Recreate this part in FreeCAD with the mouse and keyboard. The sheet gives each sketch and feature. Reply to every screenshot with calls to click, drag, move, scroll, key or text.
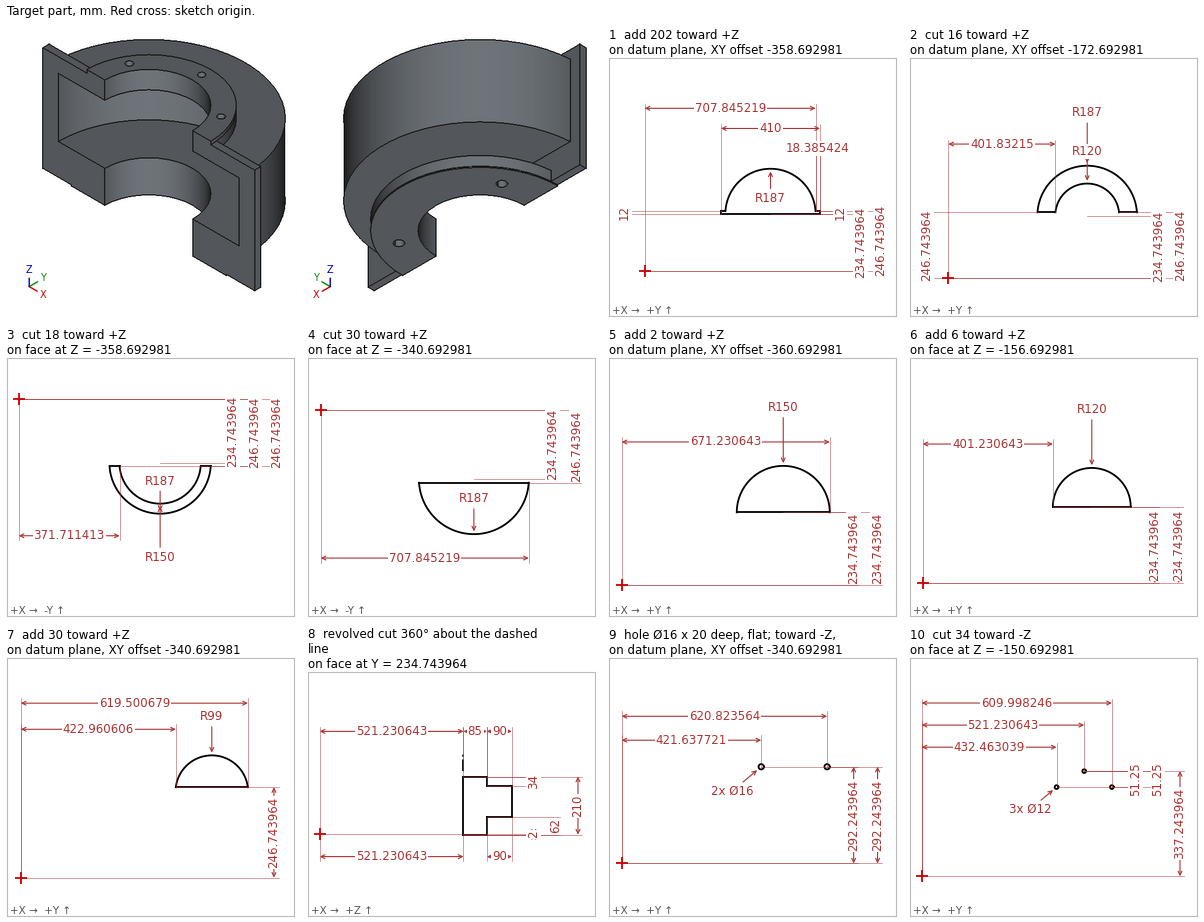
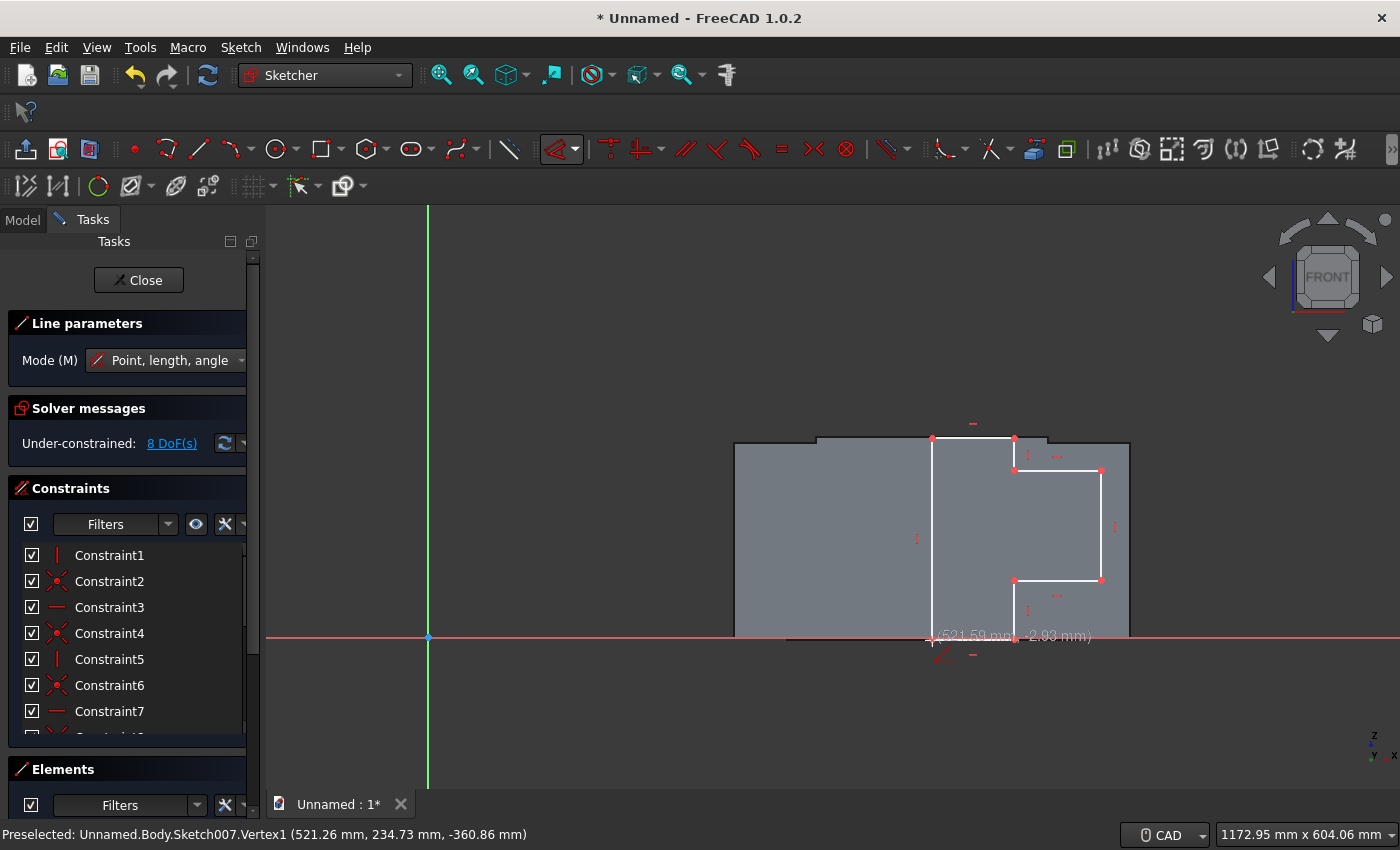
click(932, 417)
click(932, 356)
key(Escape)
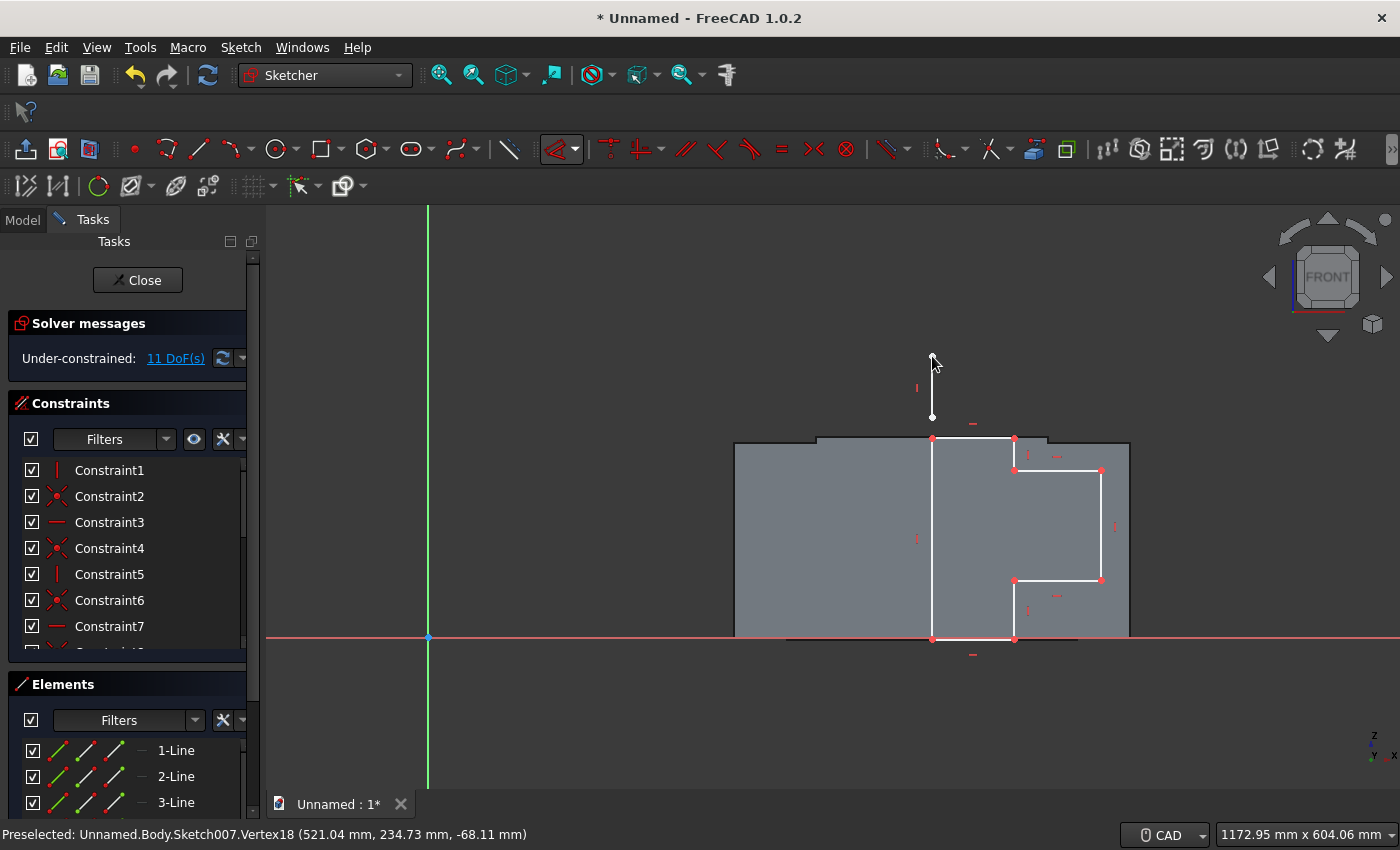
click(932, 400)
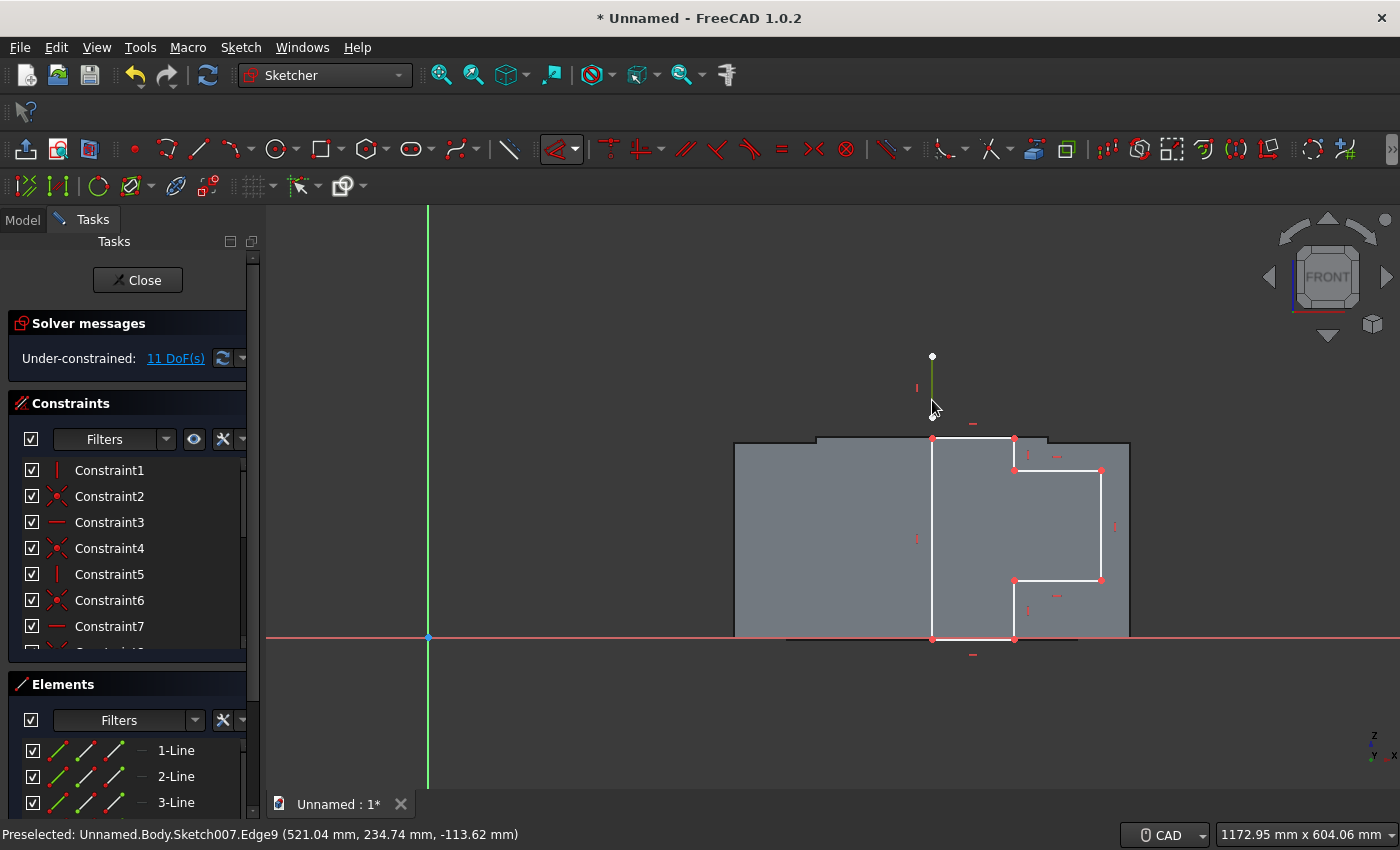
key(g)
key(n)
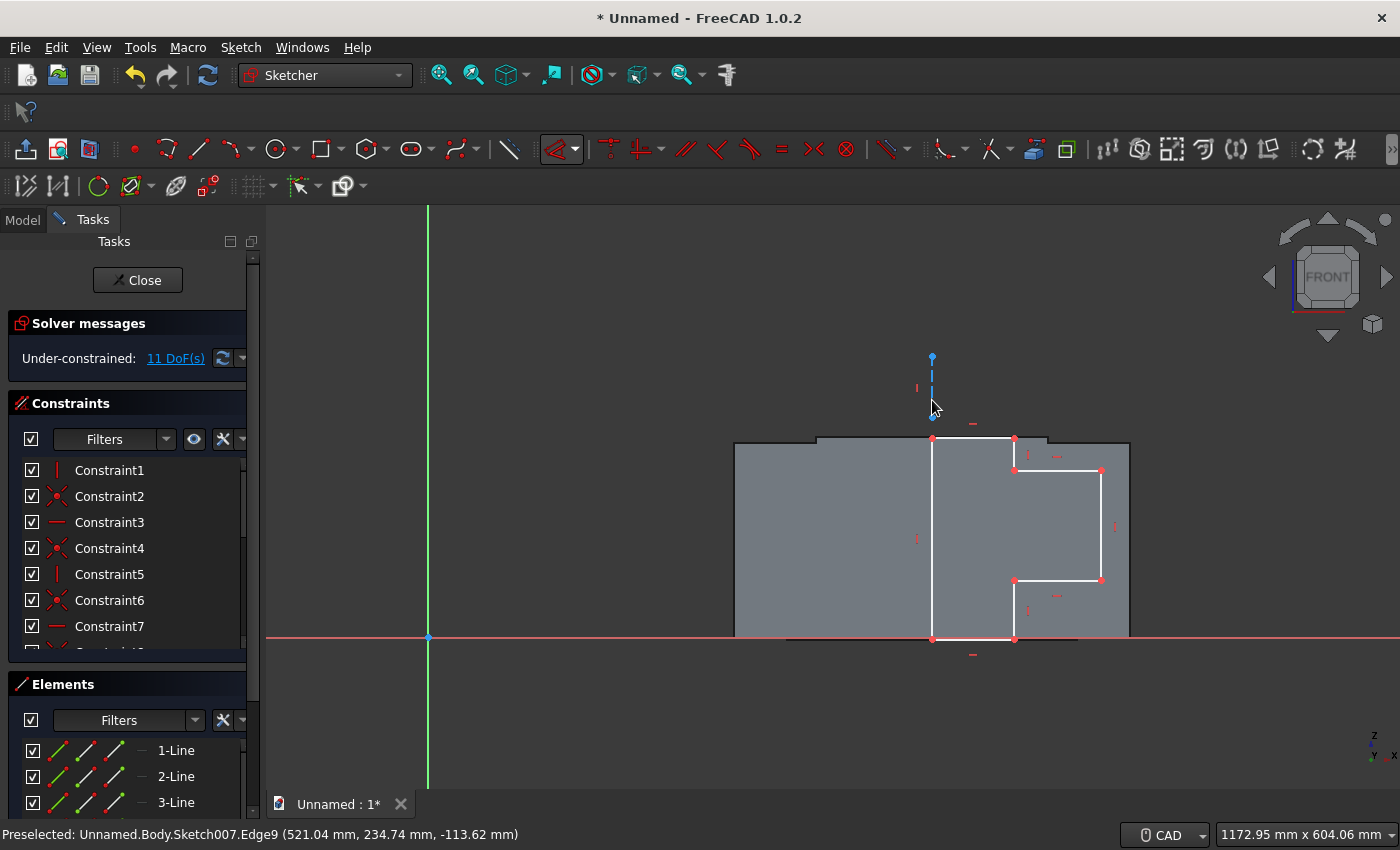
key(d)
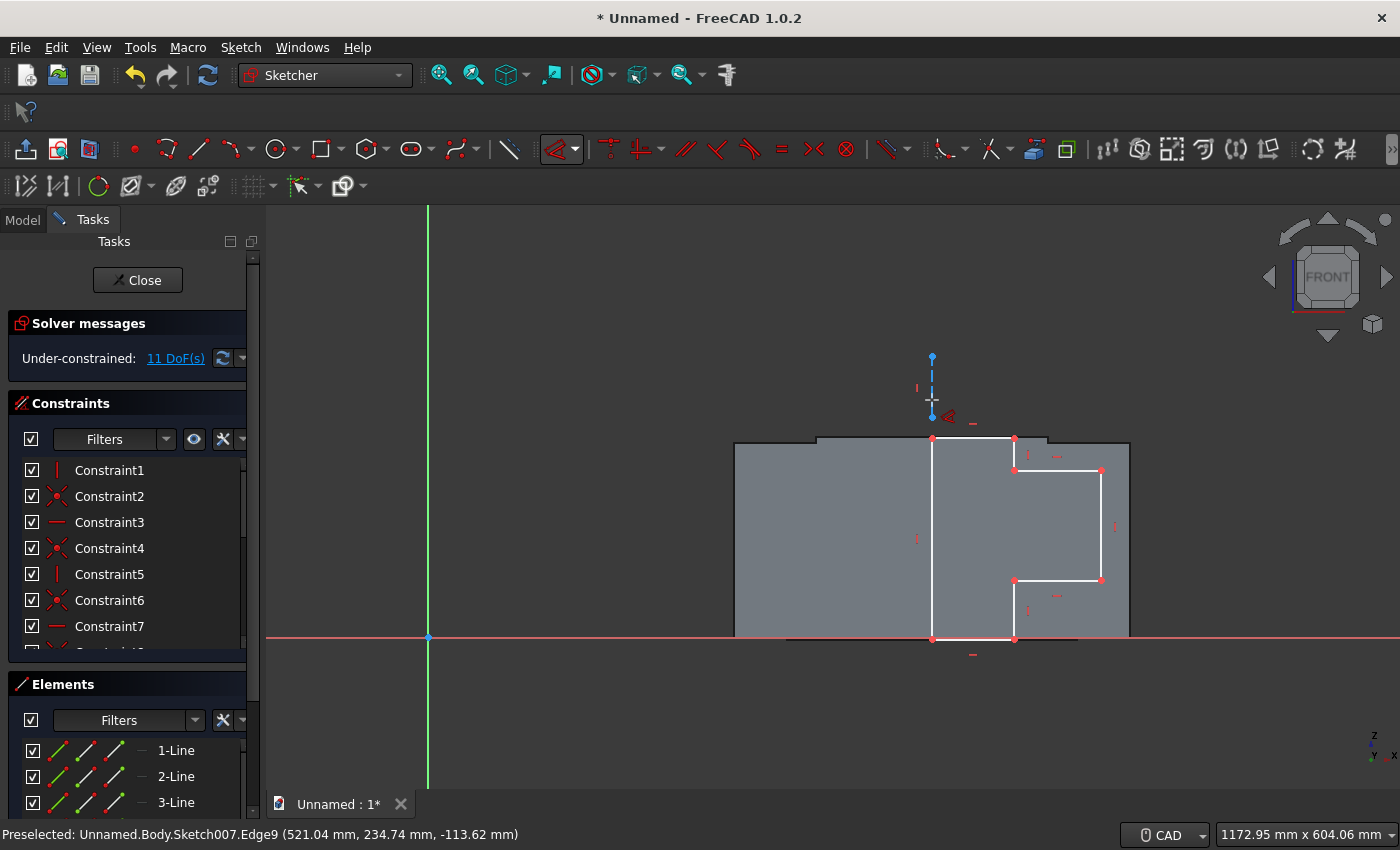
click(957, 438)
click(973, 404)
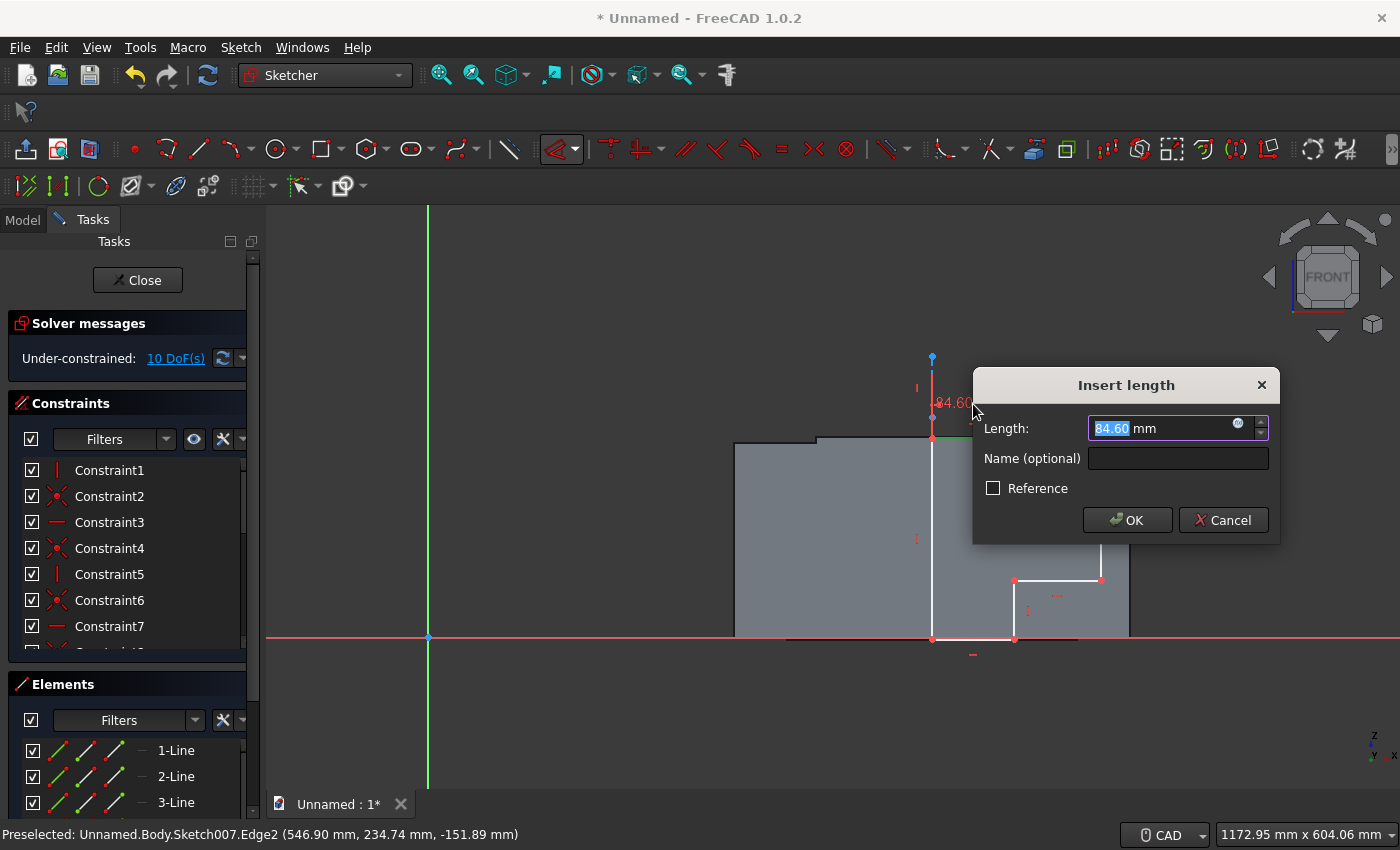
text(85)
key(Return)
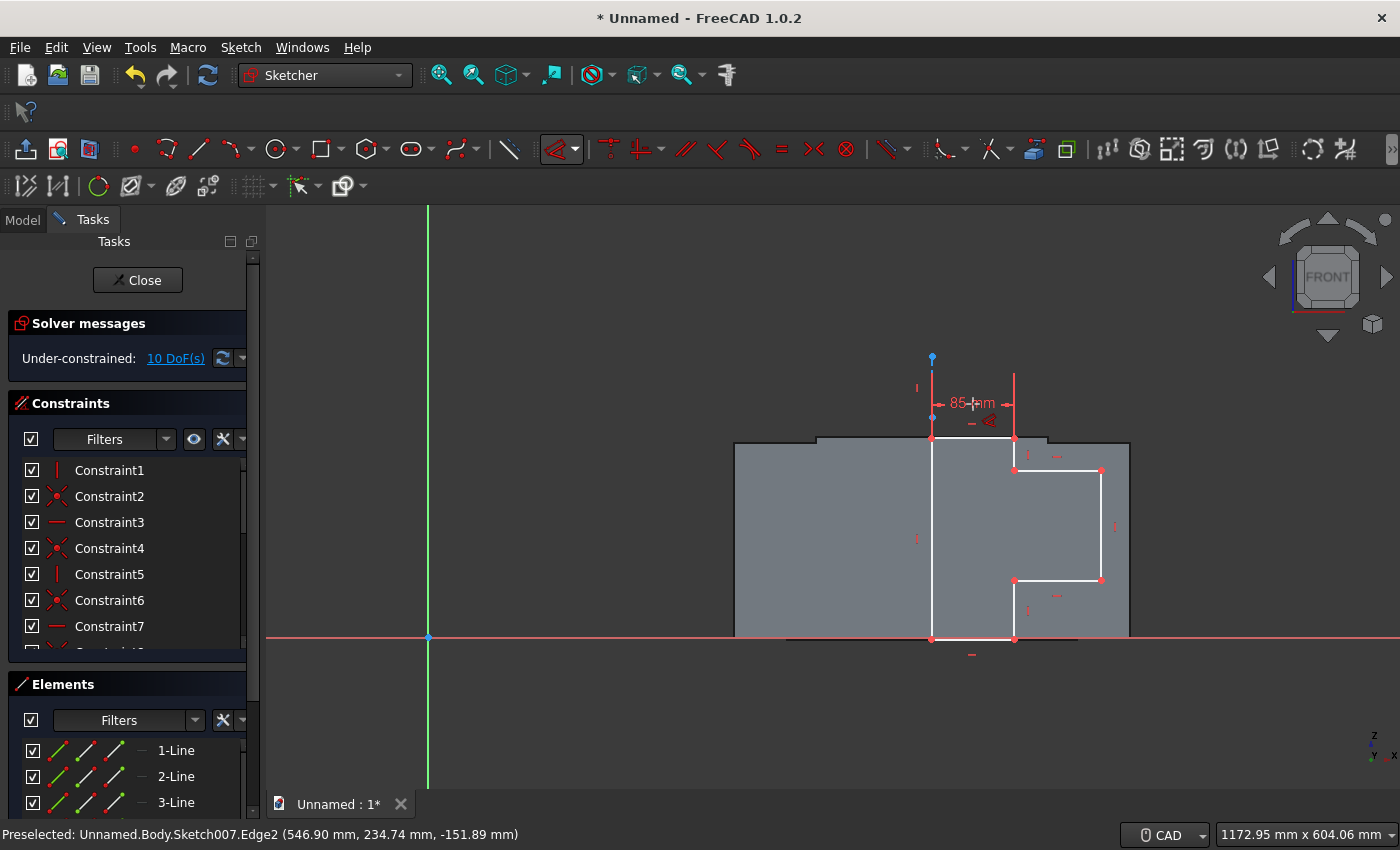
scroll(1014, 448, up, 2)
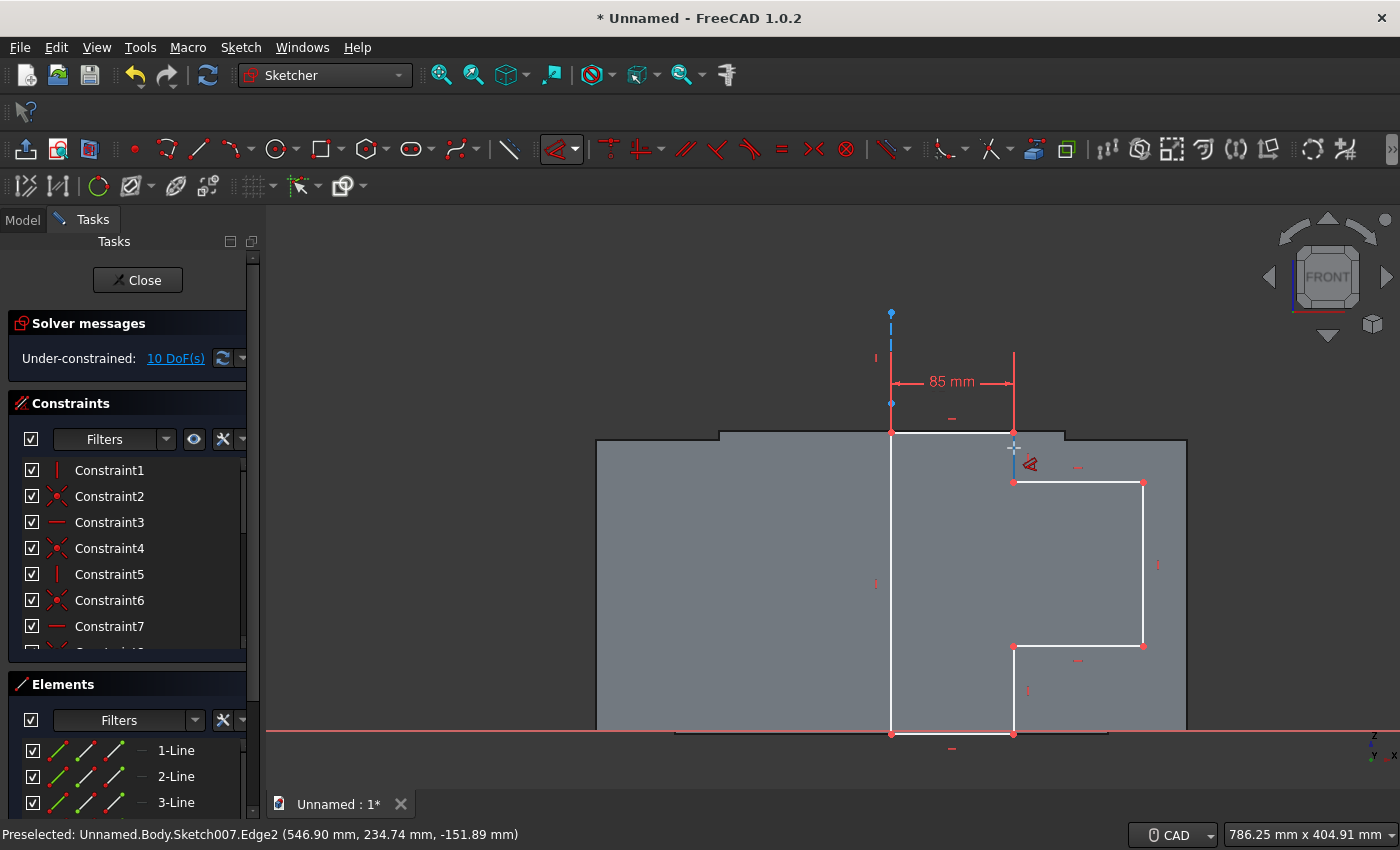
click(1014, 448)
click(1048, 457)